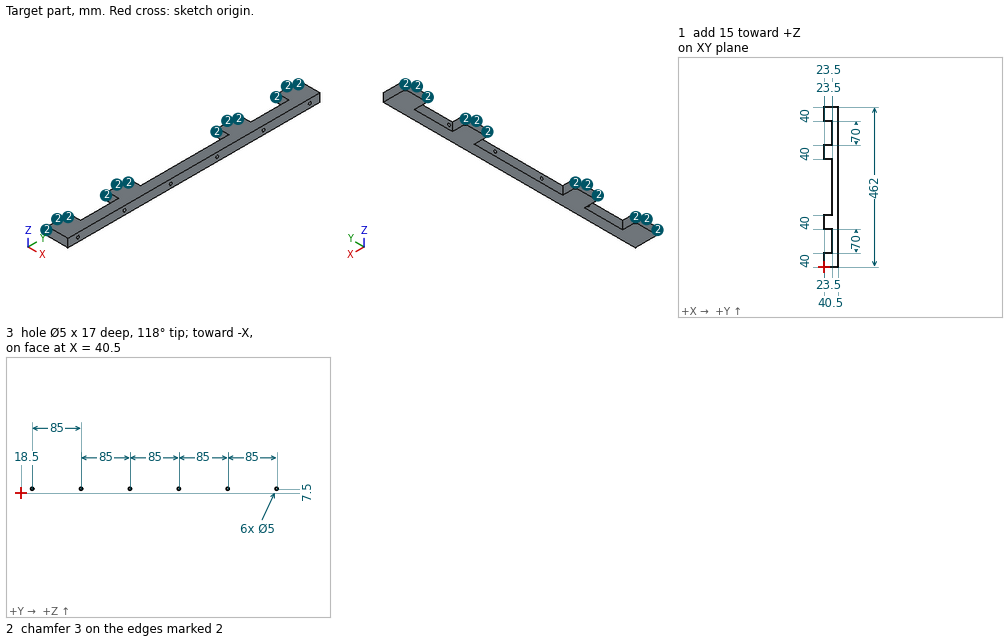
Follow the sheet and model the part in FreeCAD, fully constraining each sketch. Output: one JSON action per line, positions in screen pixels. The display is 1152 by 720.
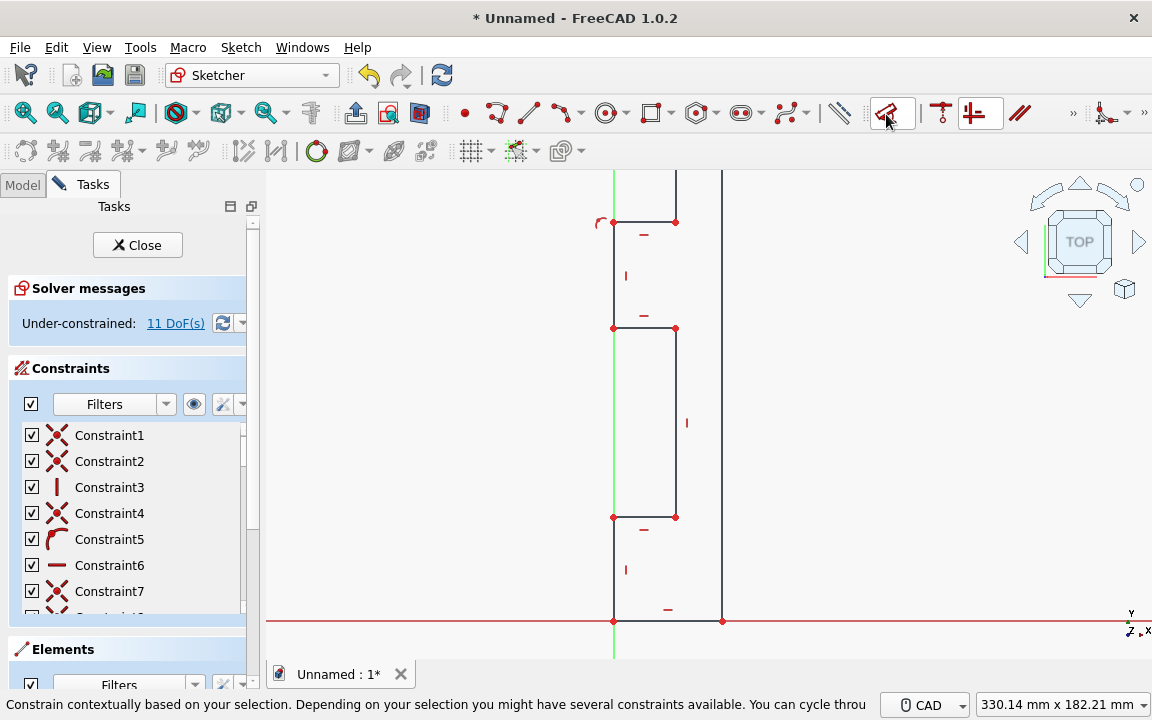
{"action": "scroll", "coordinate": [631, 550], "scroll_direction": "down", "scroll_amount": 7}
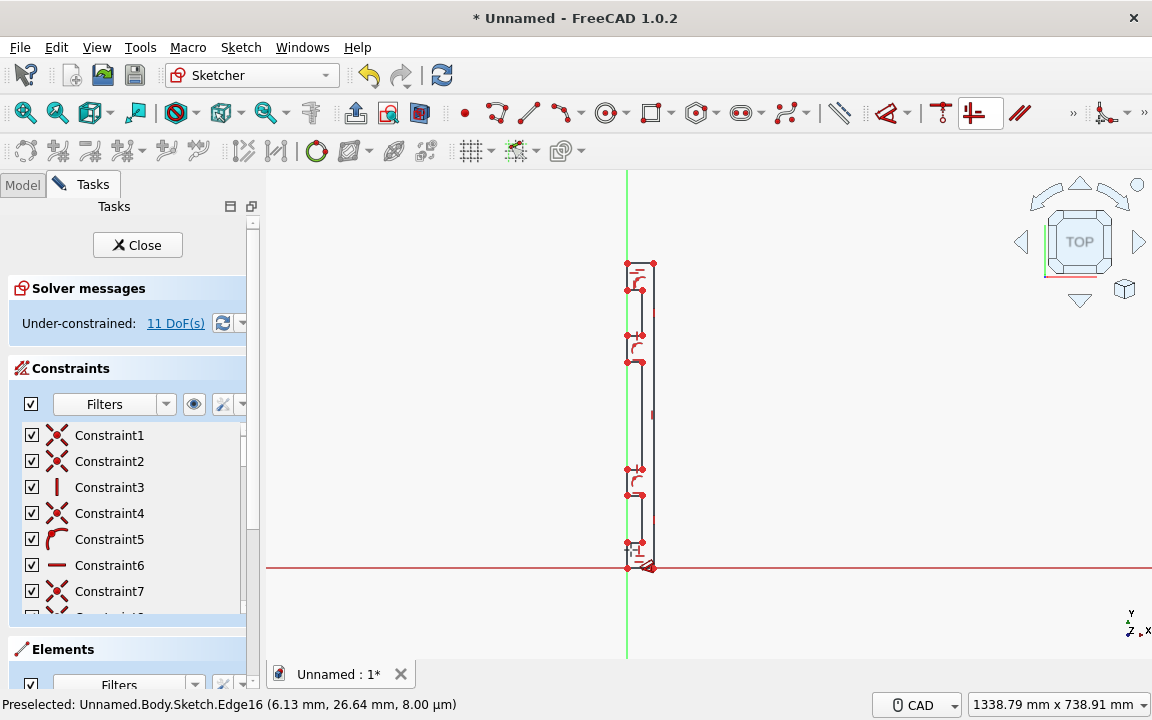
{"action": "scroll", "coordinate": [627, 271], "scroll_direction": "up", "scroll_amount": 3}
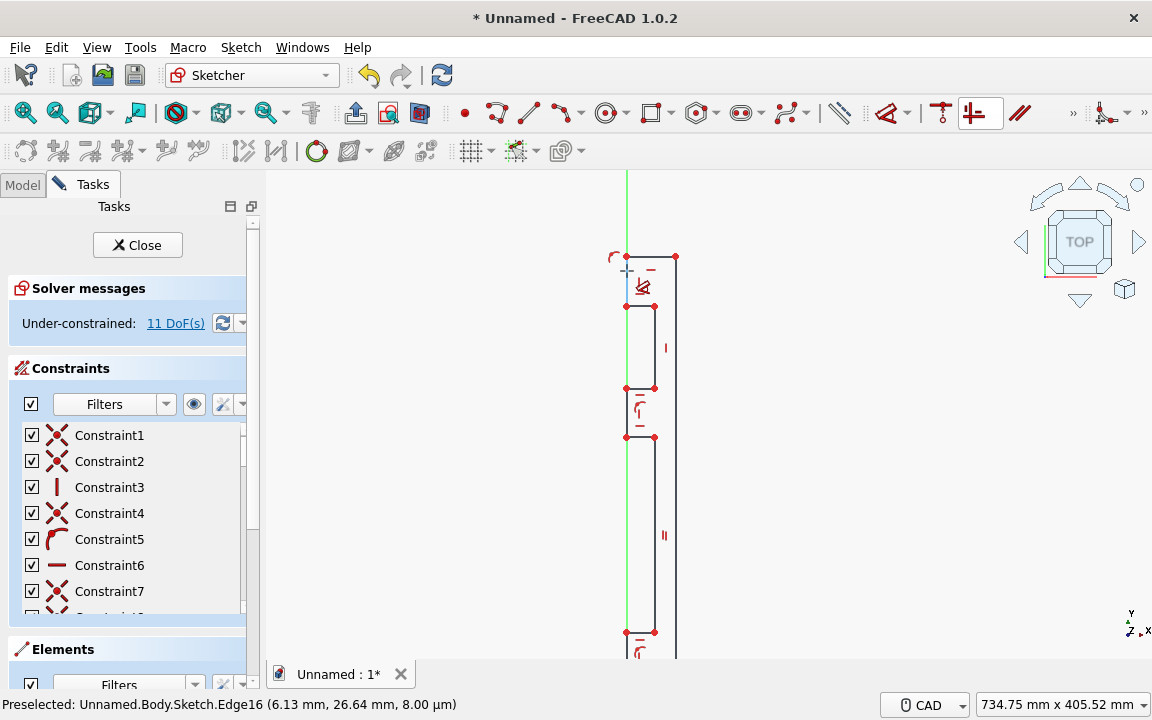
{"action": "left_click", "coordinate": [627, 272]}
{"action": "left_click", "coordinate": [593, 281]}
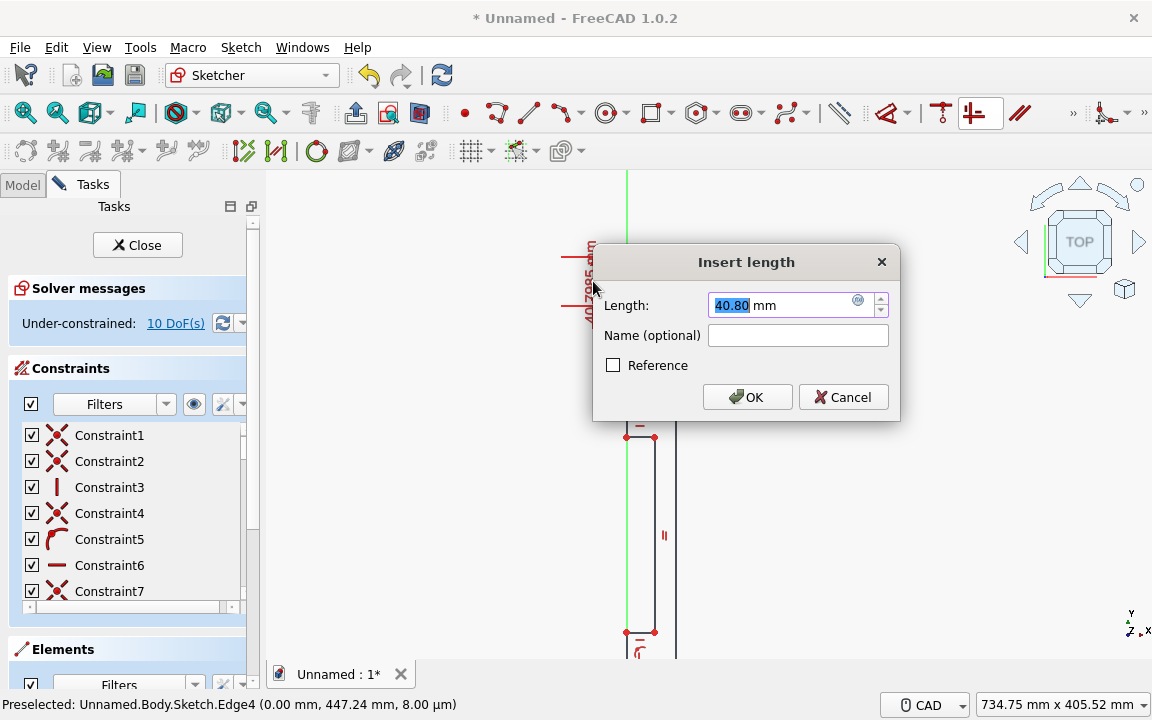
{"action": "type", "text": "40"}
{"action": "key", "text": "Return"}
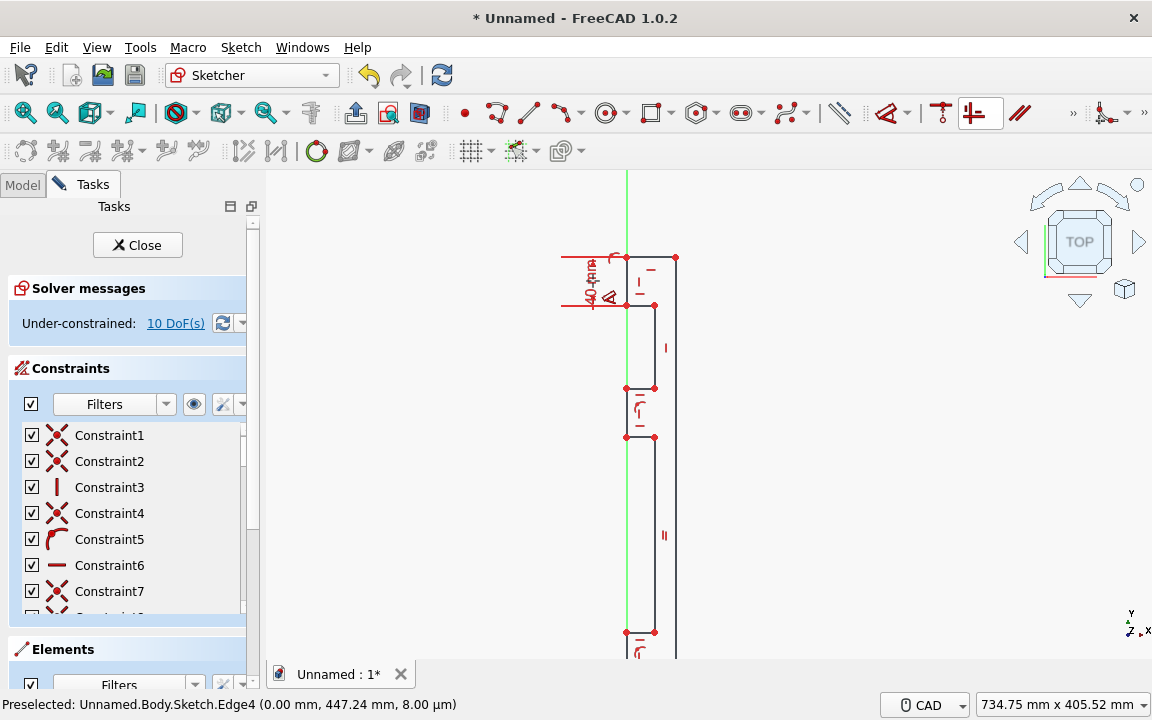
{"action": "left_click", "coordinate": [655, 331]}
{"action": "left_click", "coordinate": [713, 347]}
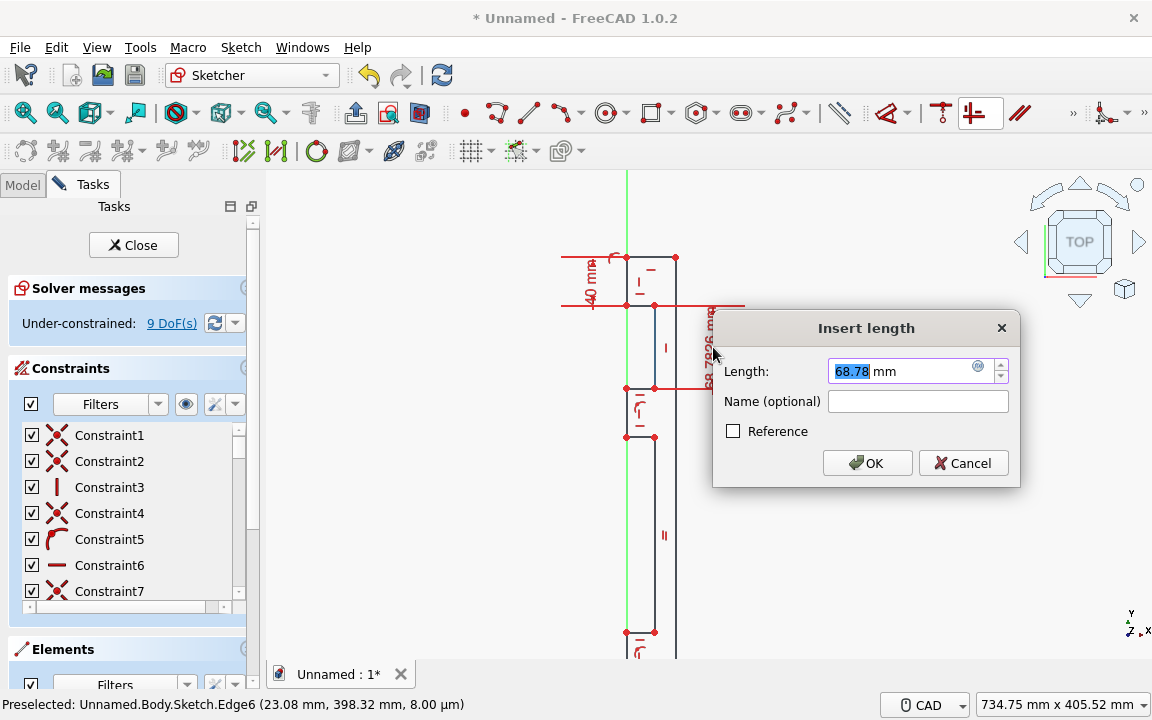
{"action": "type", "text": "70"}
{"action": "key", "text": "Return"}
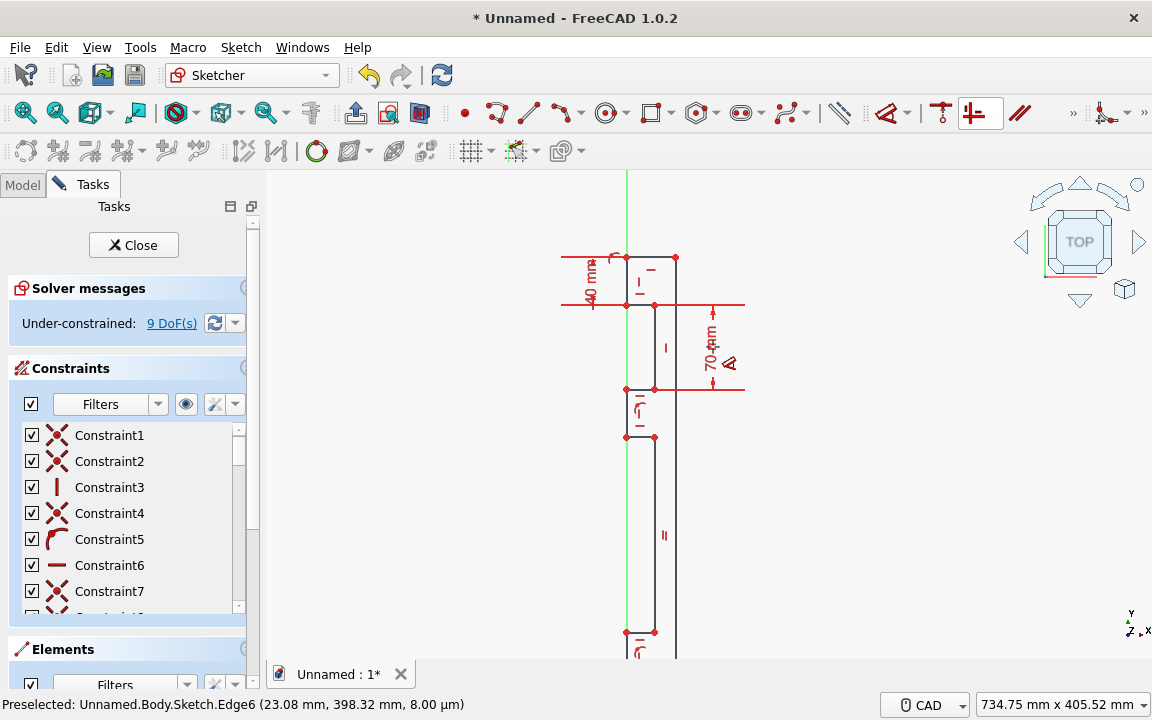
{"action": "left_click", "coordinate": [627, 404]}
{"action": "left_click", "coordinate": [593, 414]}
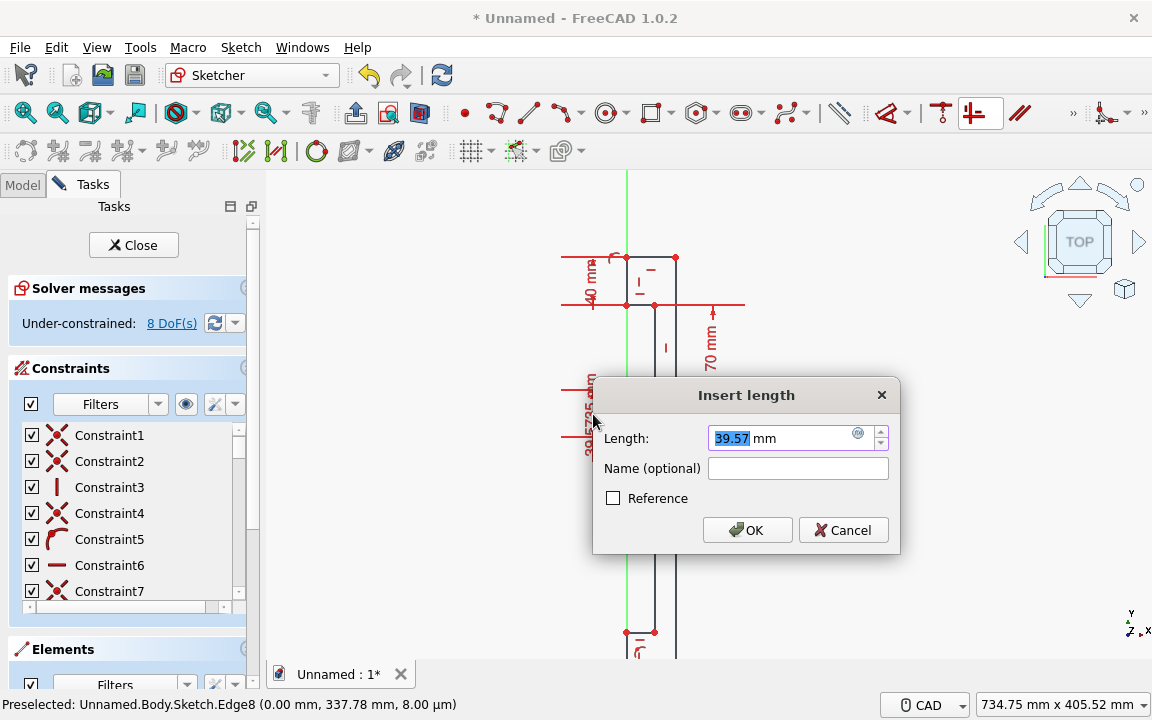
{"action": "type", "text": "40"}
{"action": "key", "text": "Return"}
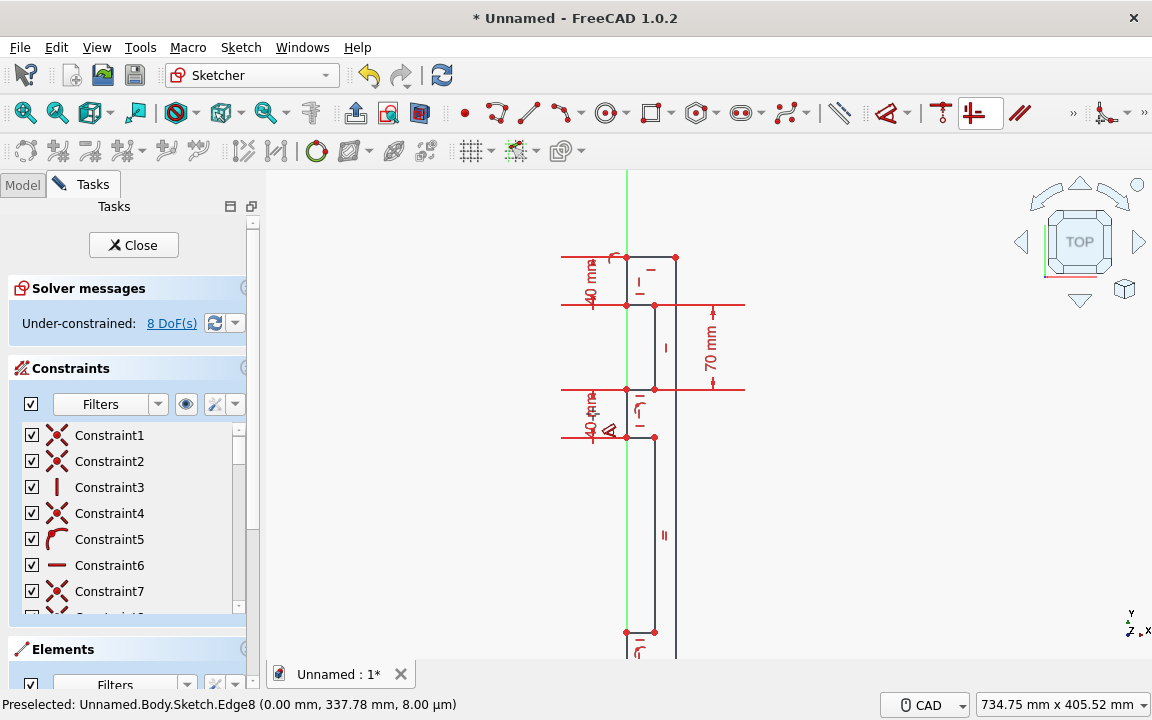
{"action": "scroll", "coordinate": [627, 269], "scroll_direction": "down", "scroll_amount": 3}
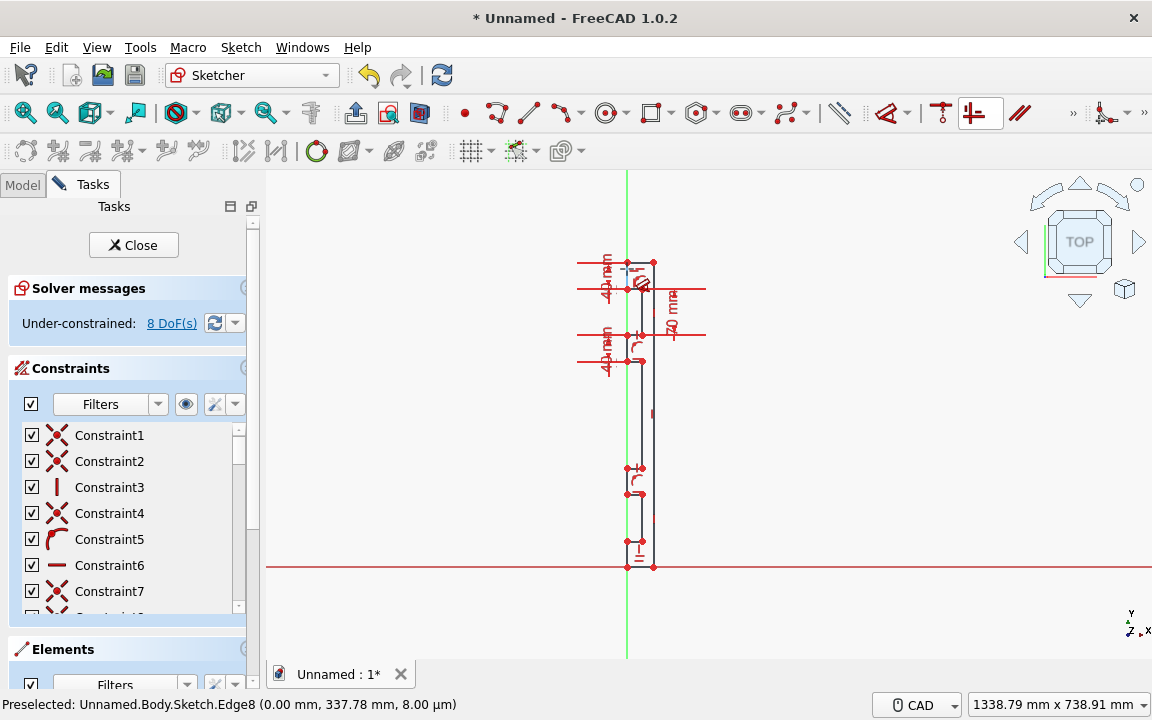
{"action": "scroll", "coordinate": [627, 477], "scroll_direction": "up", "scroll_amount": 3}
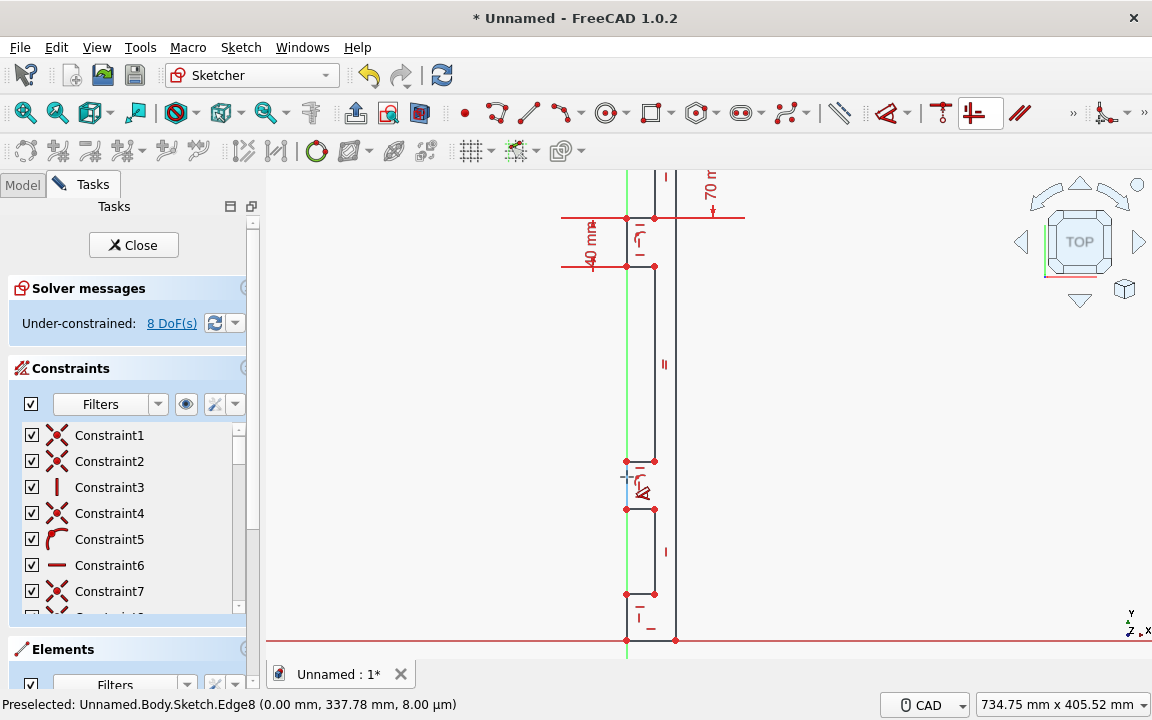
{"action": "left_click", "coordinate": [627, 476]}
{"action": "left_click", "coordinate": [593, 485]}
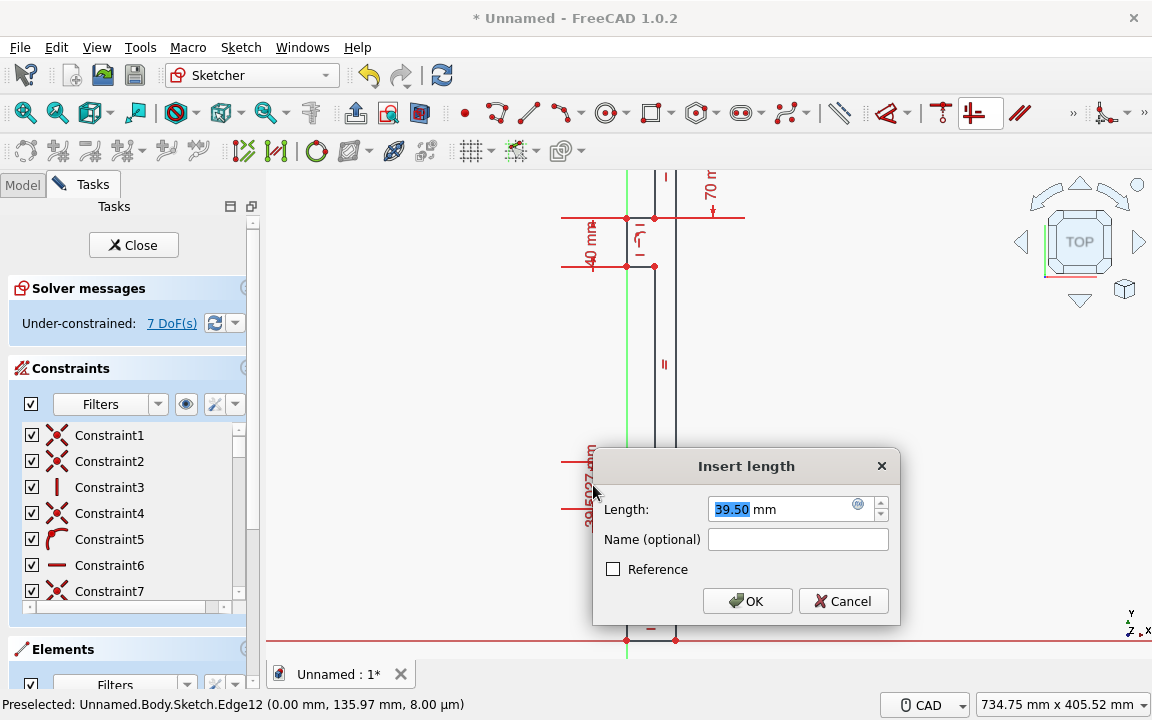
{"action": "type", "text": "40"}
{"action": "key", "text": "Return"}